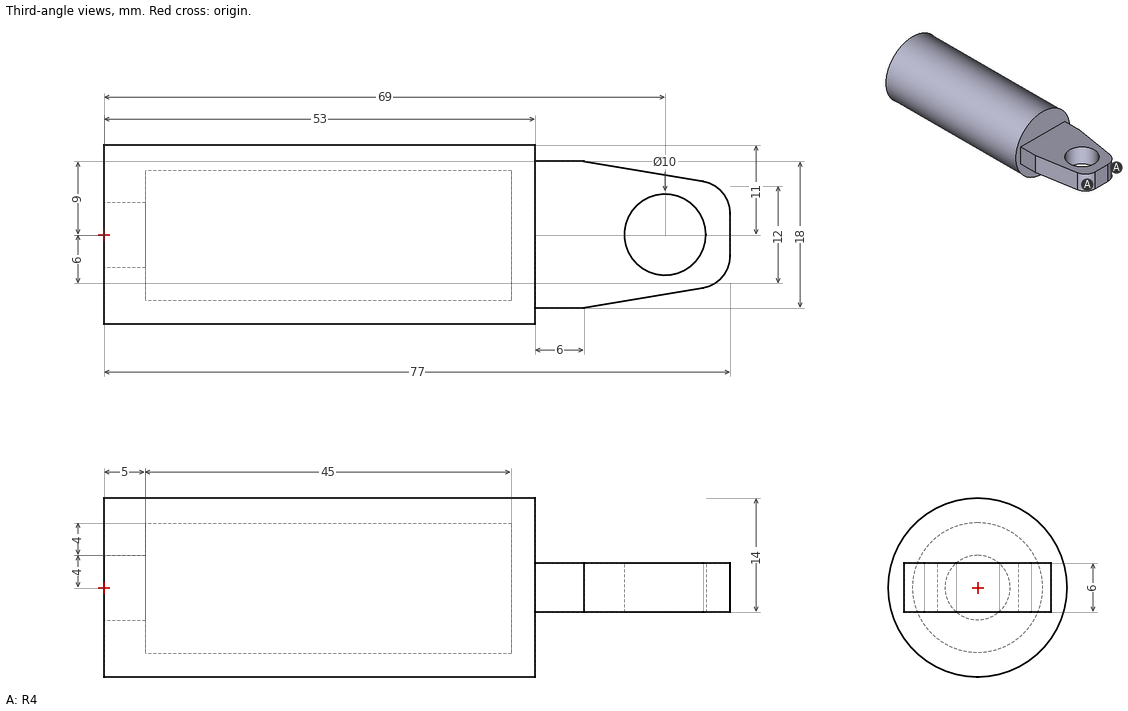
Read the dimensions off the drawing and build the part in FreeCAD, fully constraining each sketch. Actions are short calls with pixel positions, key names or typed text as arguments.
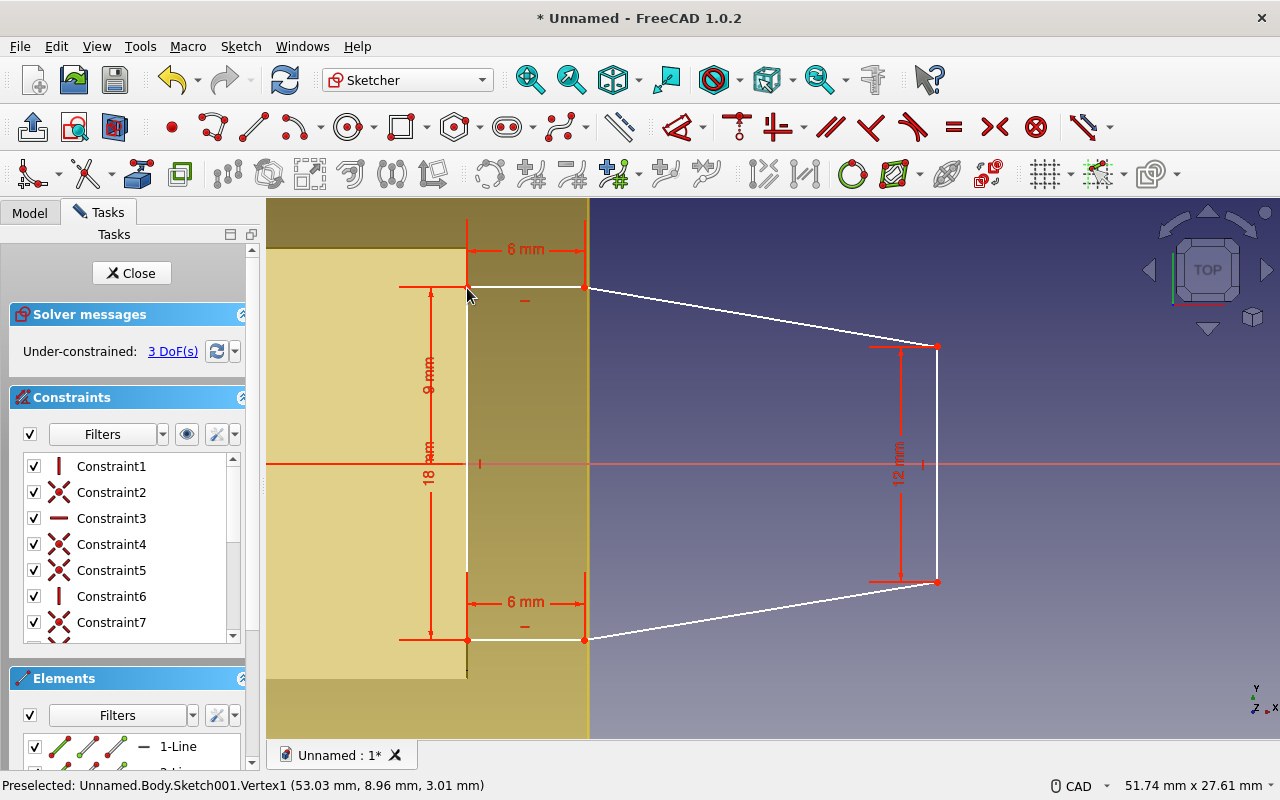
click(937, 582)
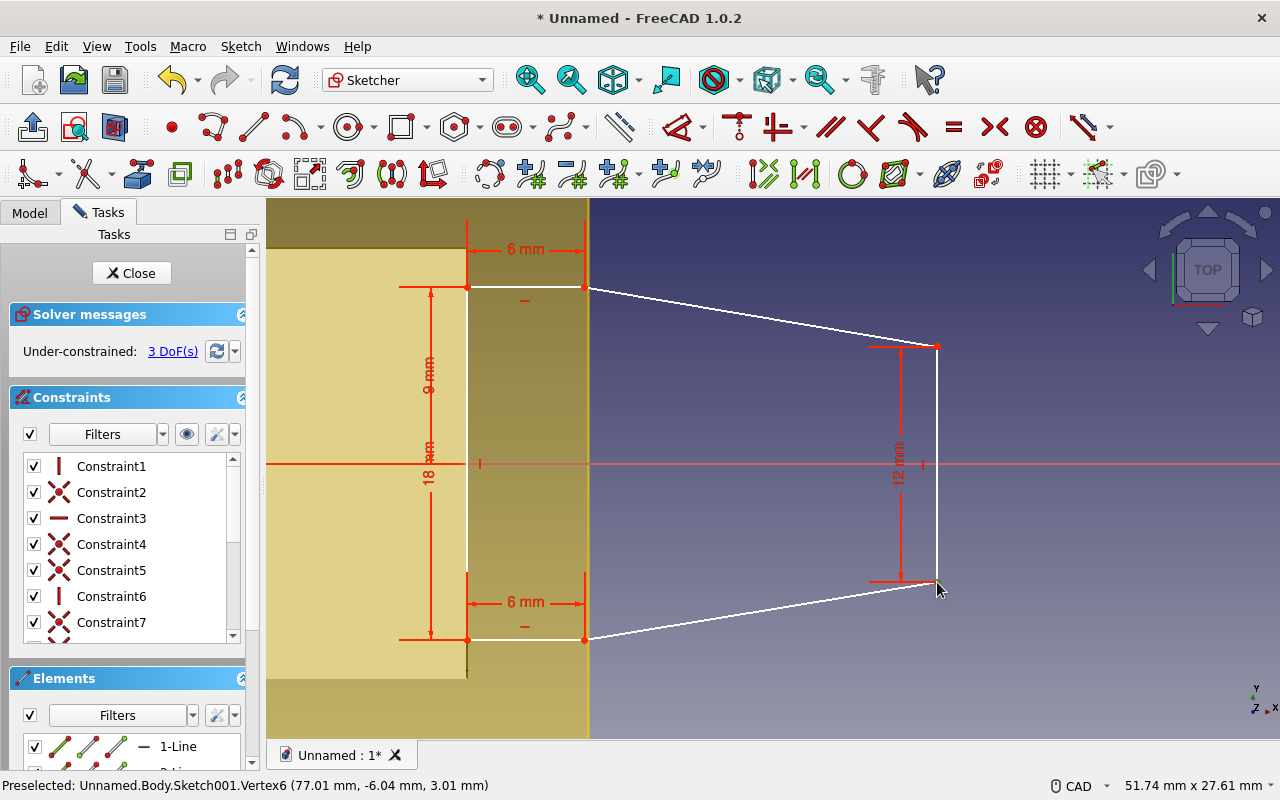
key(i)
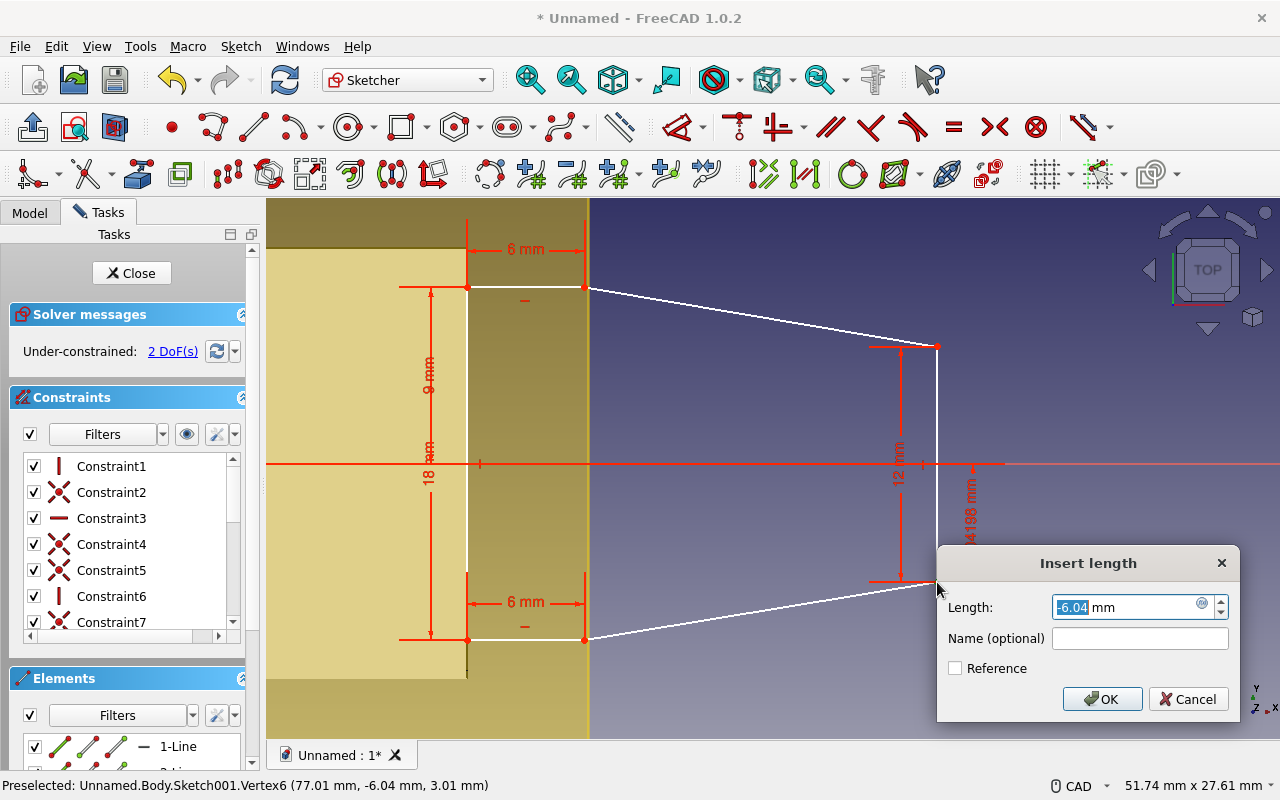
text(-6)
key(Return)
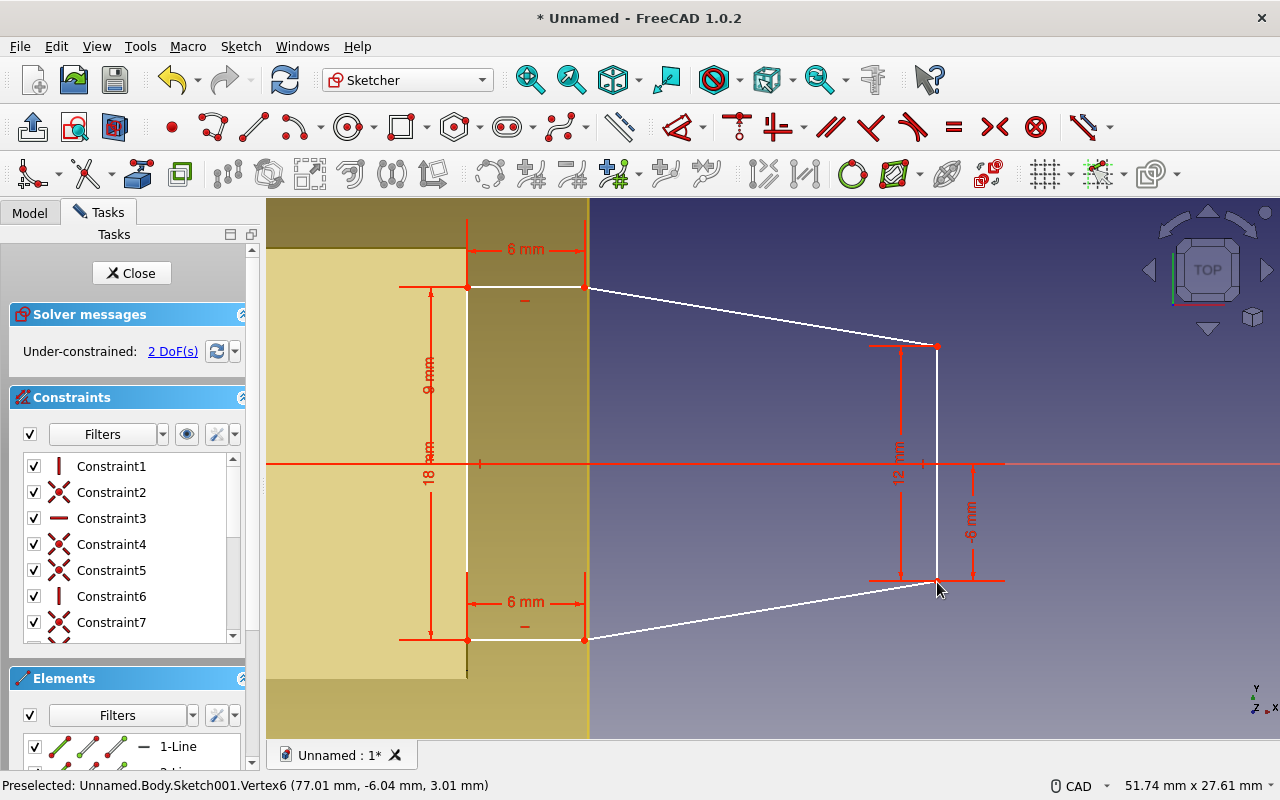
click(467, 287)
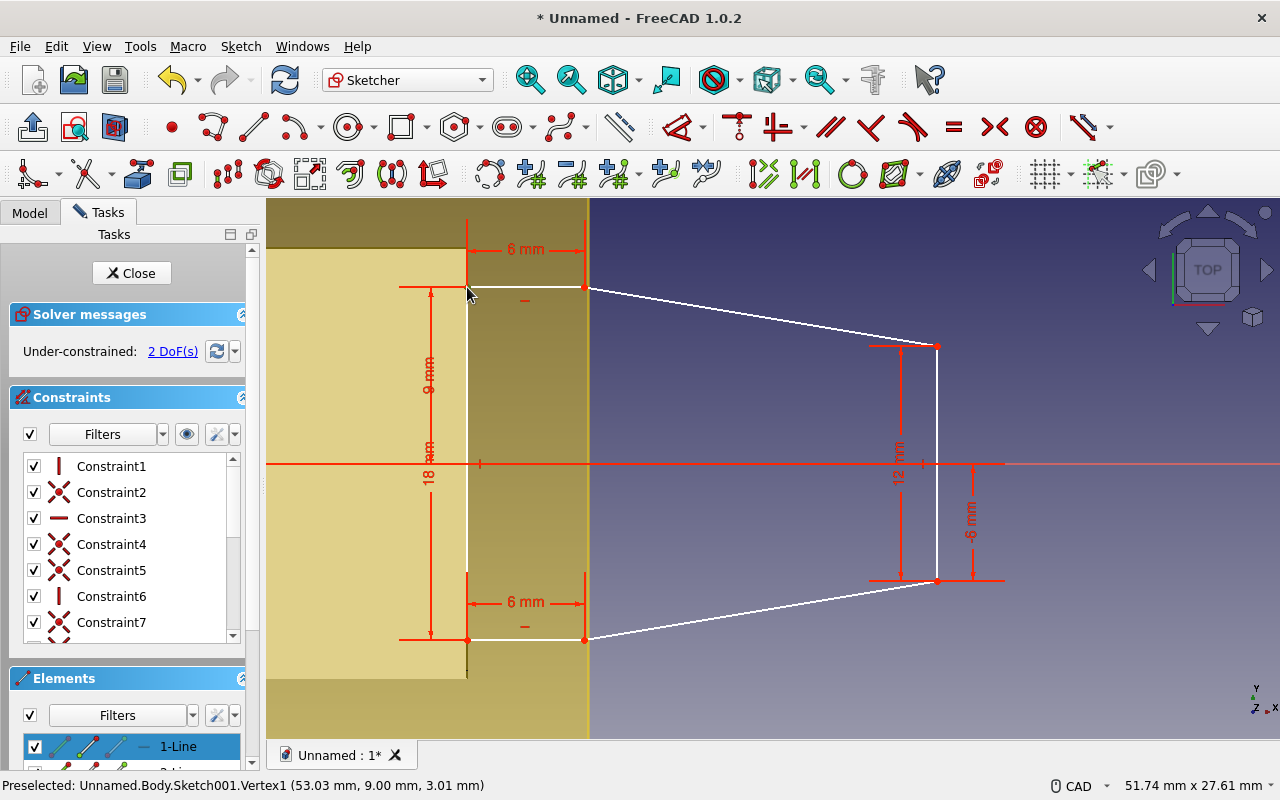
key(l)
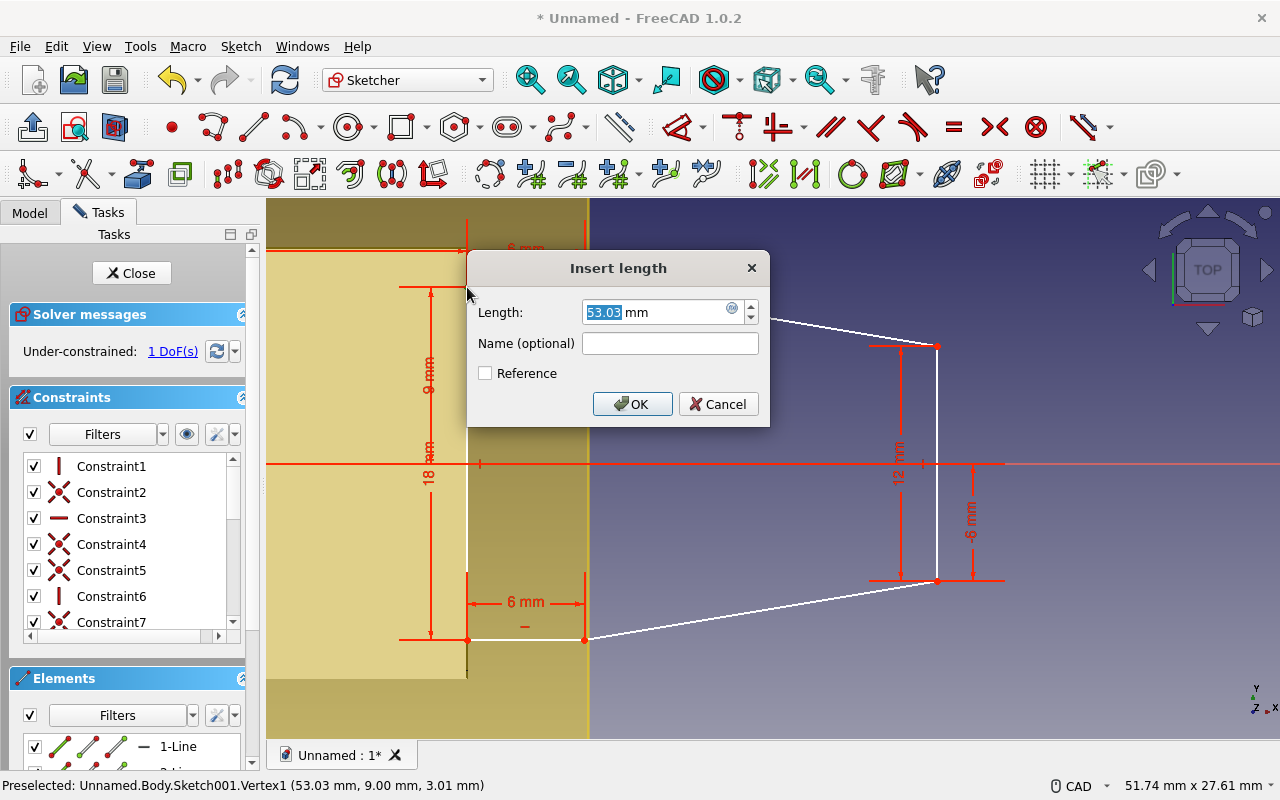
text(53)
key(Return)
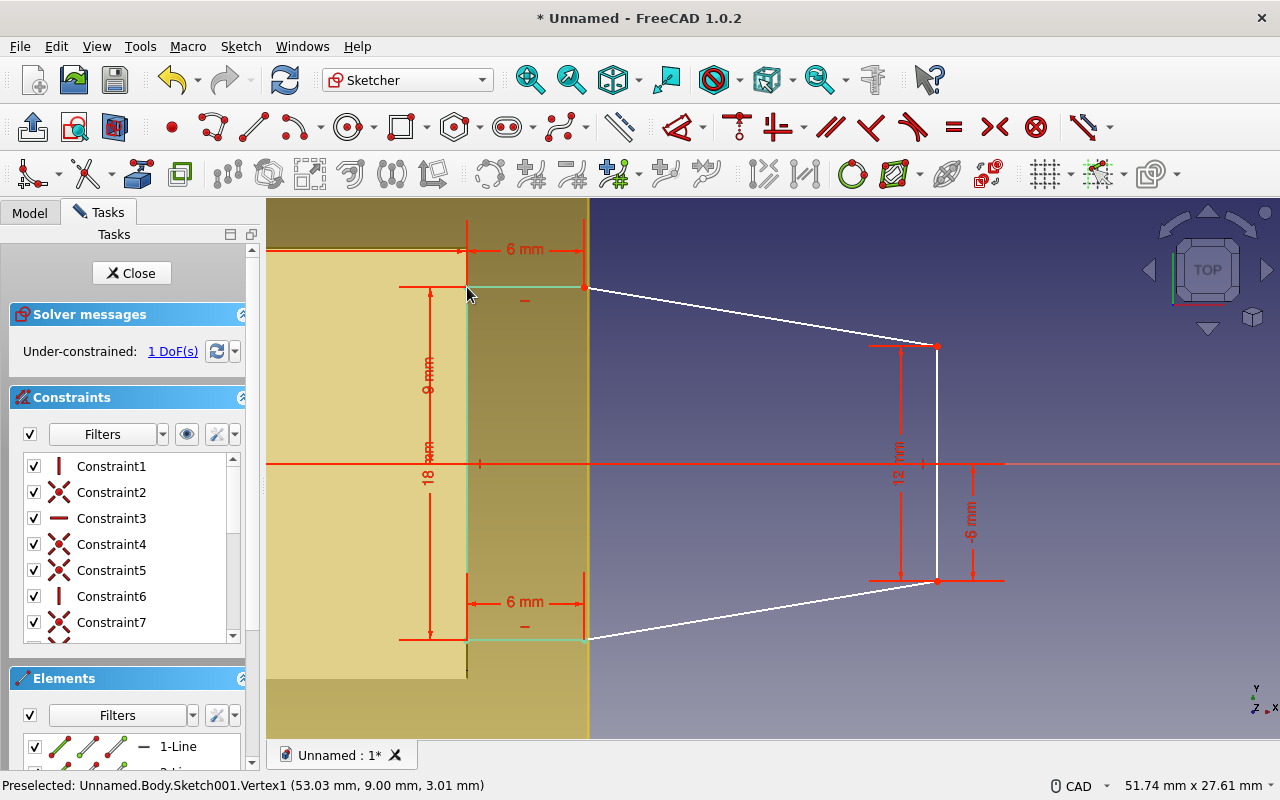
click(937, 581)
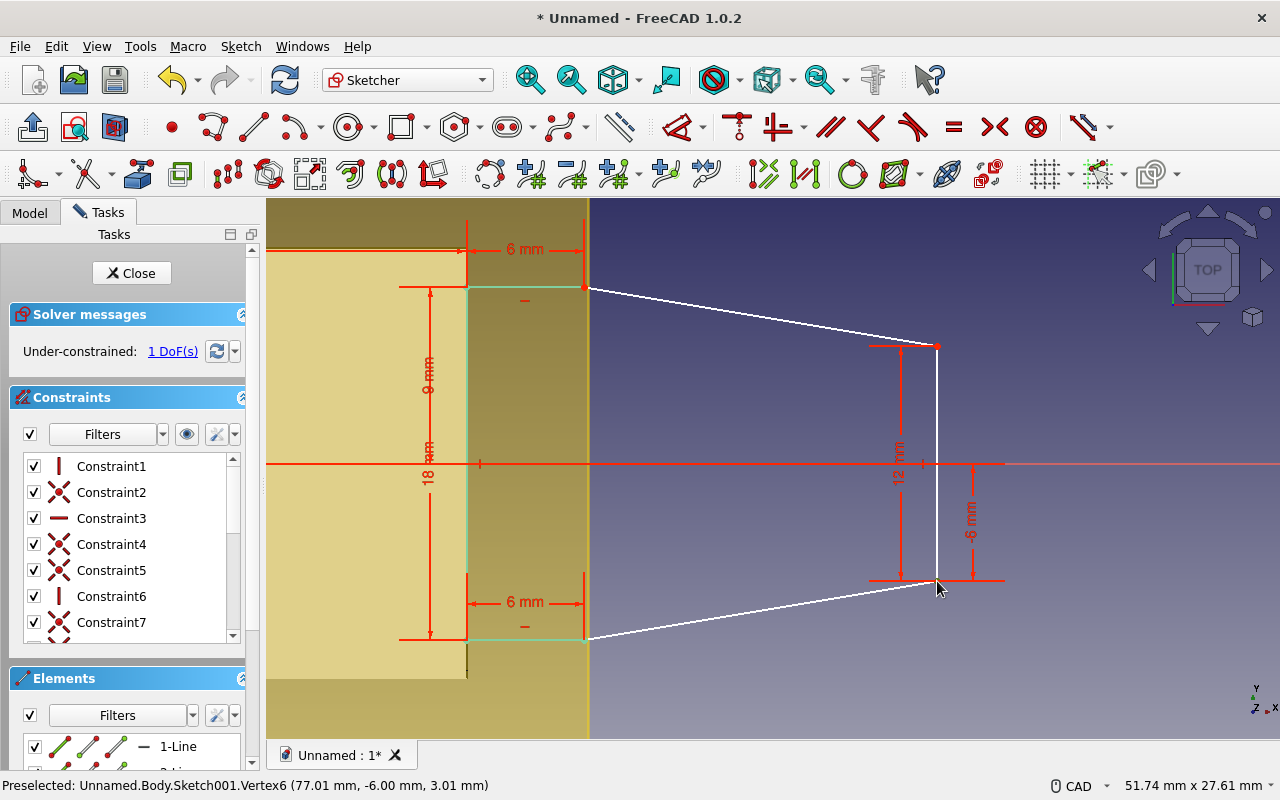
key(l)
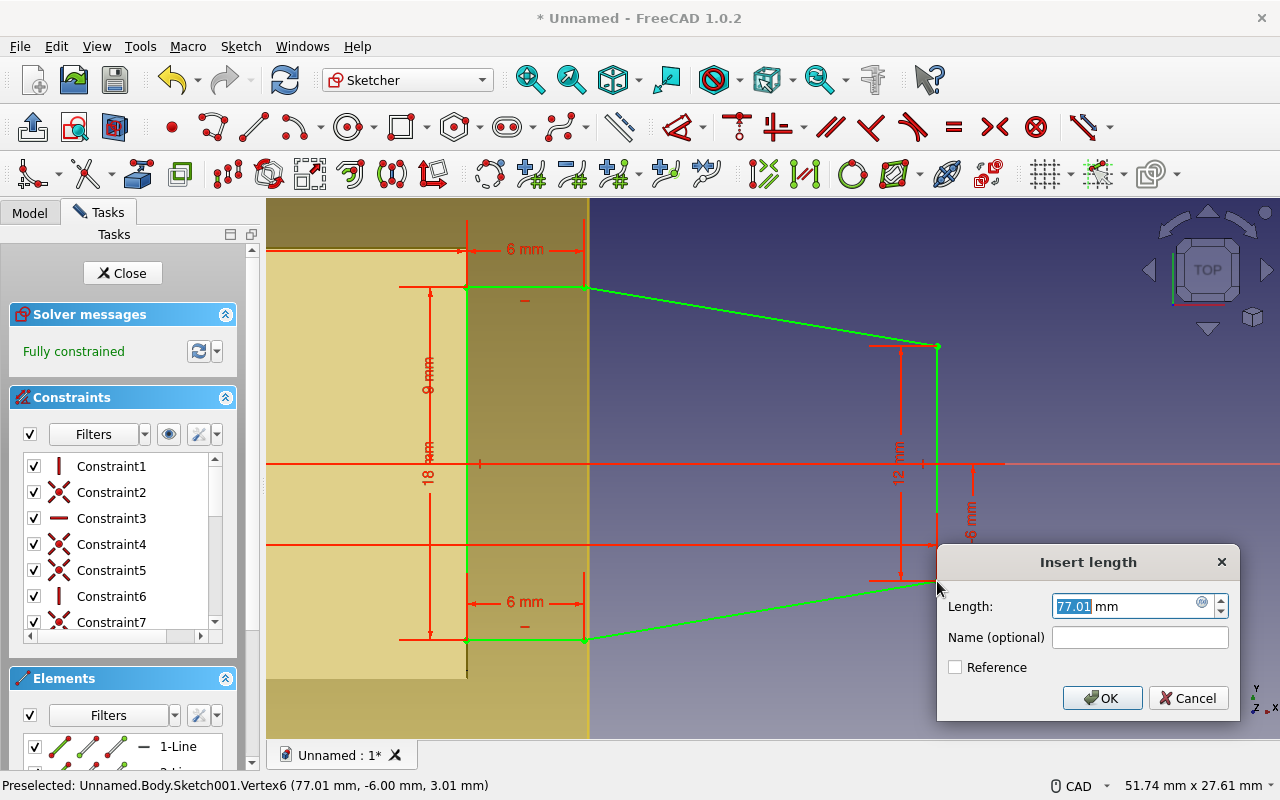
text(77)
key(Return)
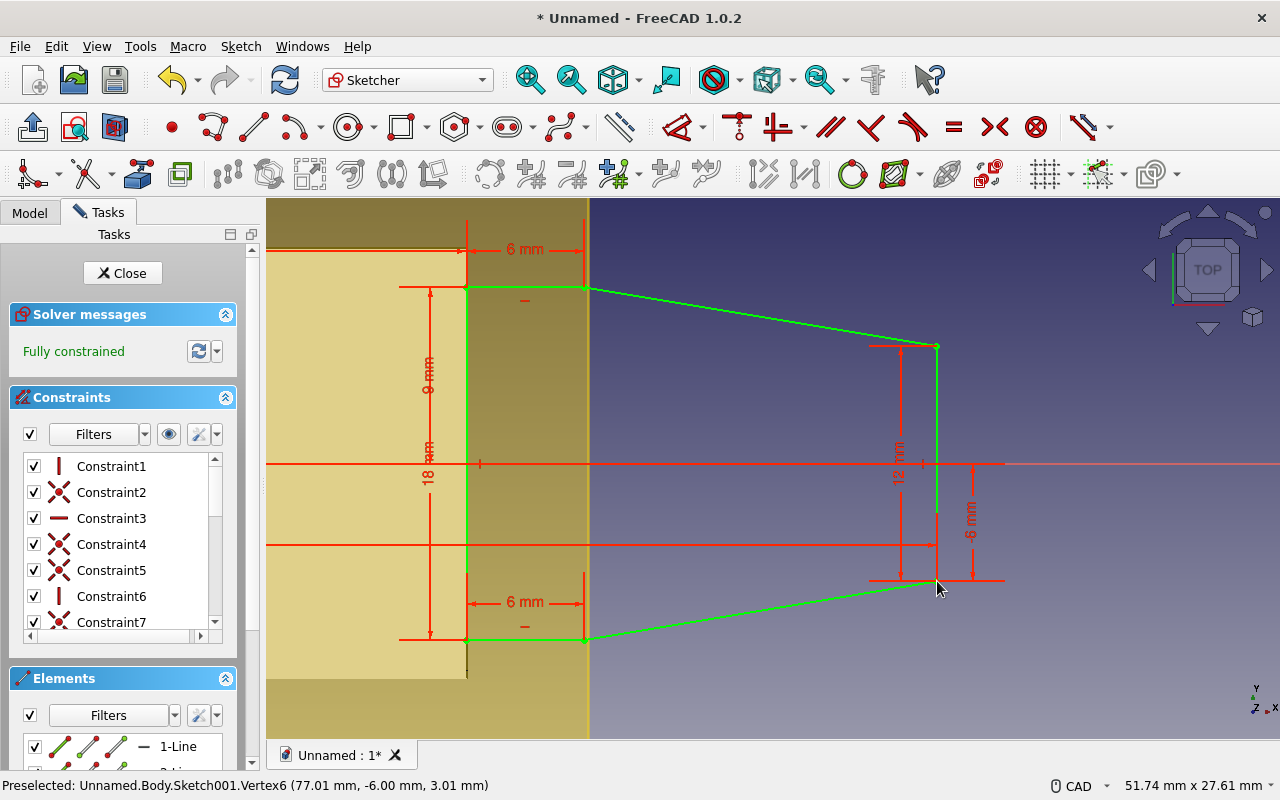
click(123, 273)